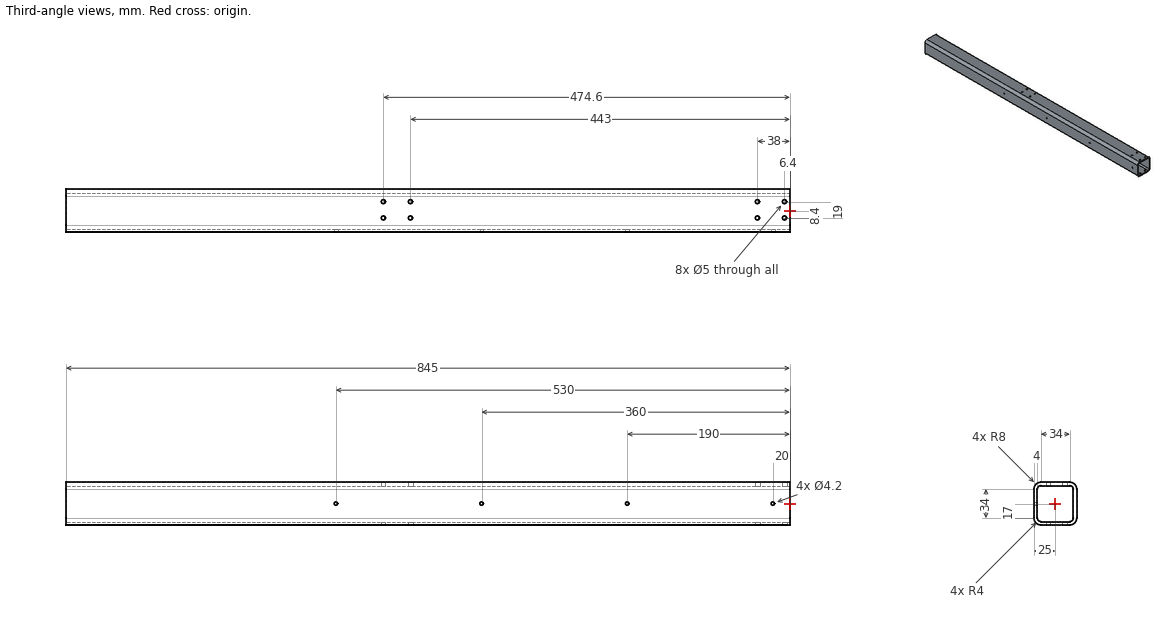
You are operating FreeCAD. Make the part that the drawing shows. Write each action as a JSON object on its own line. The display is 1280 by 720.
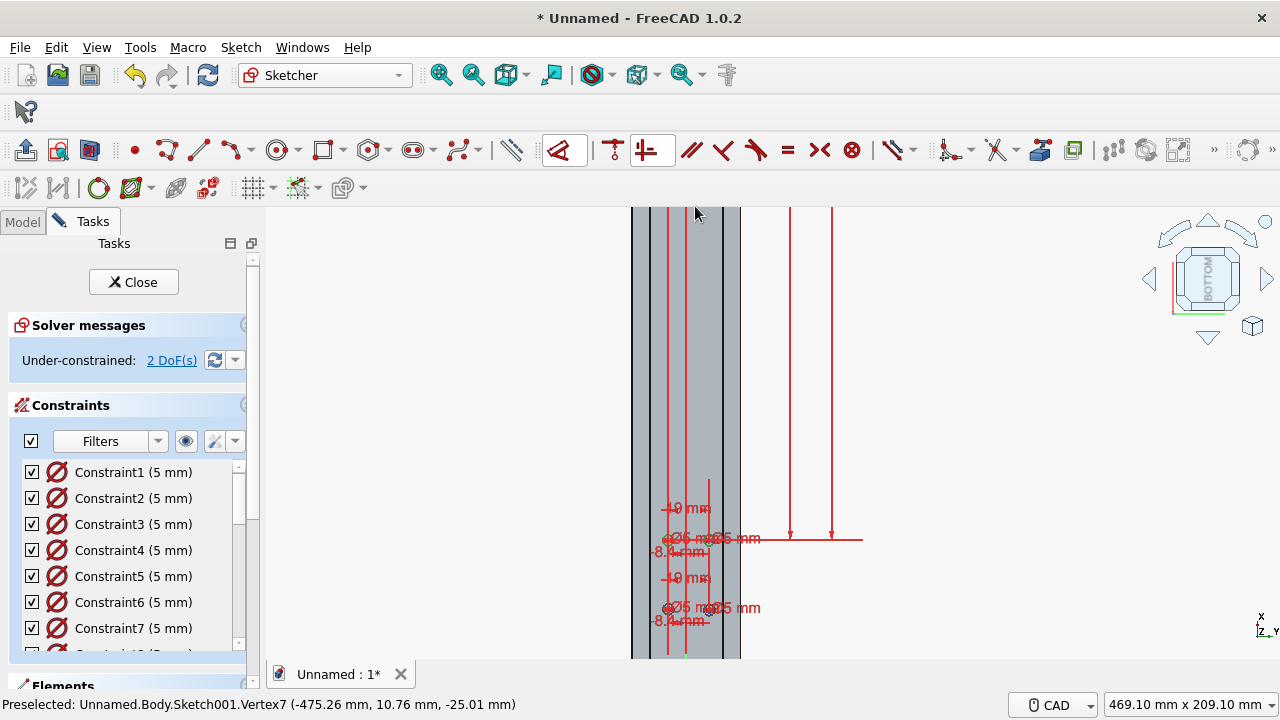
{"action": "scroll", "coordinate": [710, 542], "scroll_direction": "down", "scroll_amount": 7}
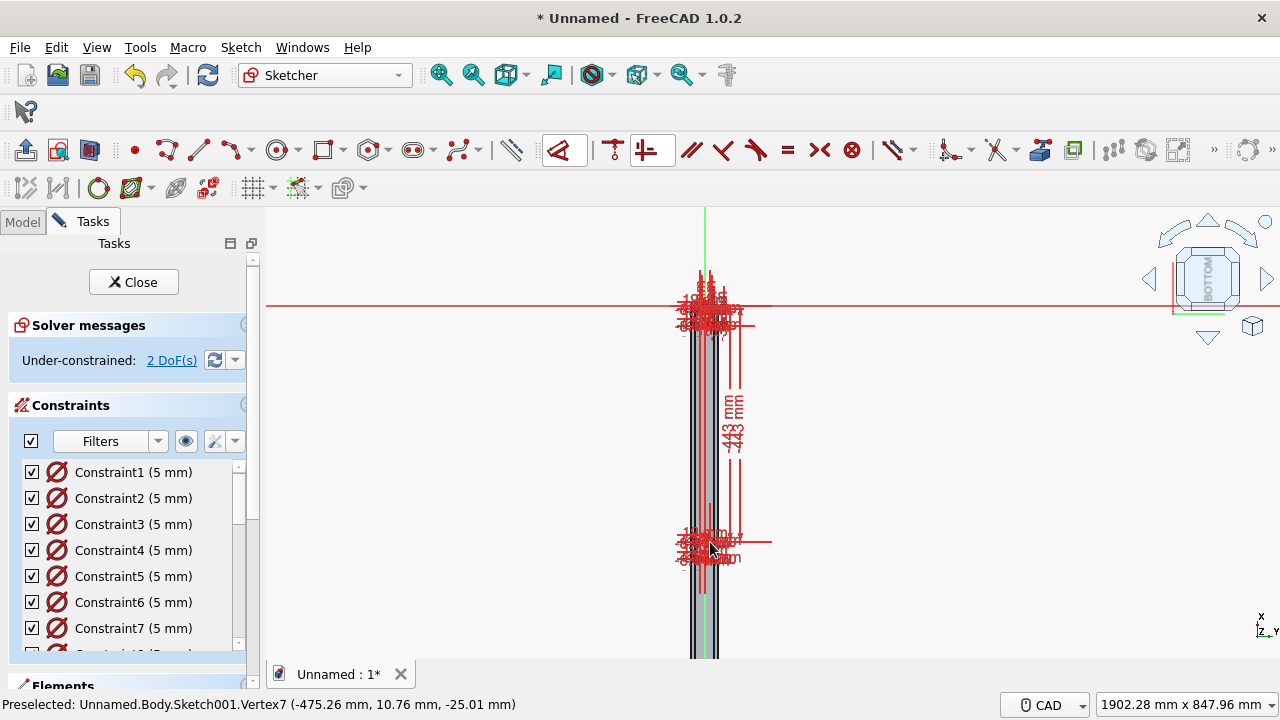
{"action": "left_click", "coordinate": [710, 559]}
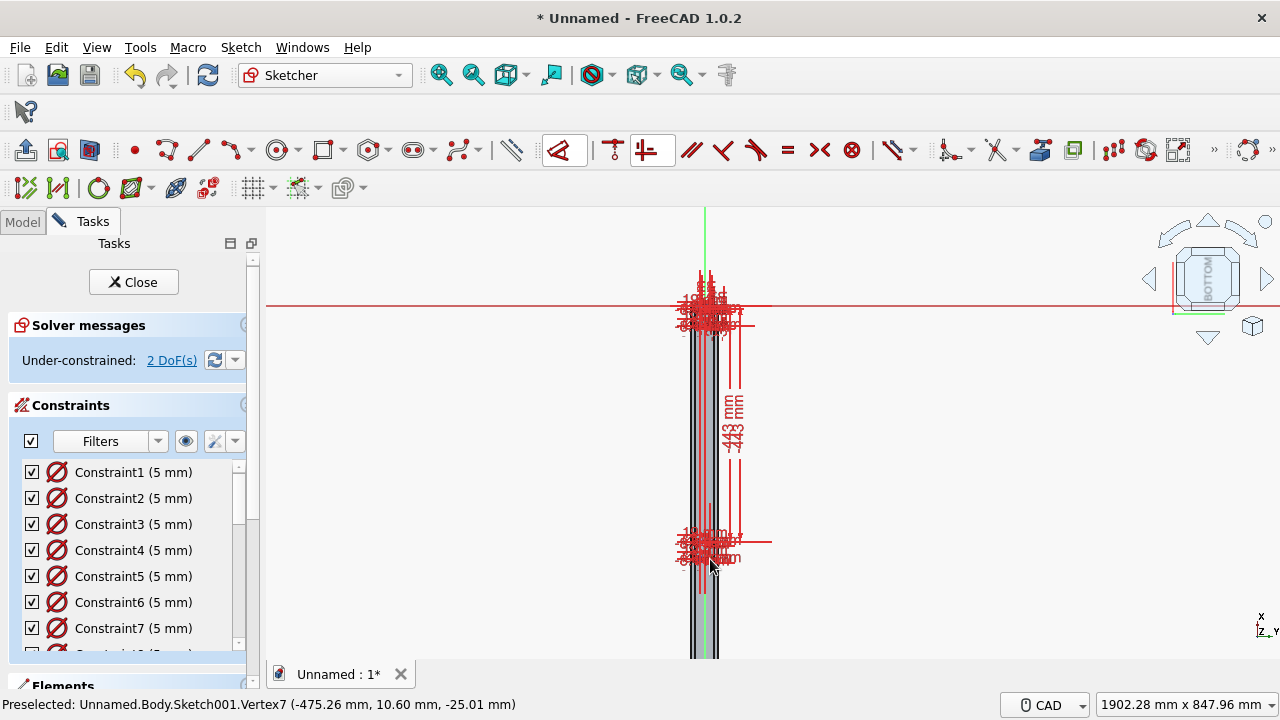
{"action": "key", "text": "i"}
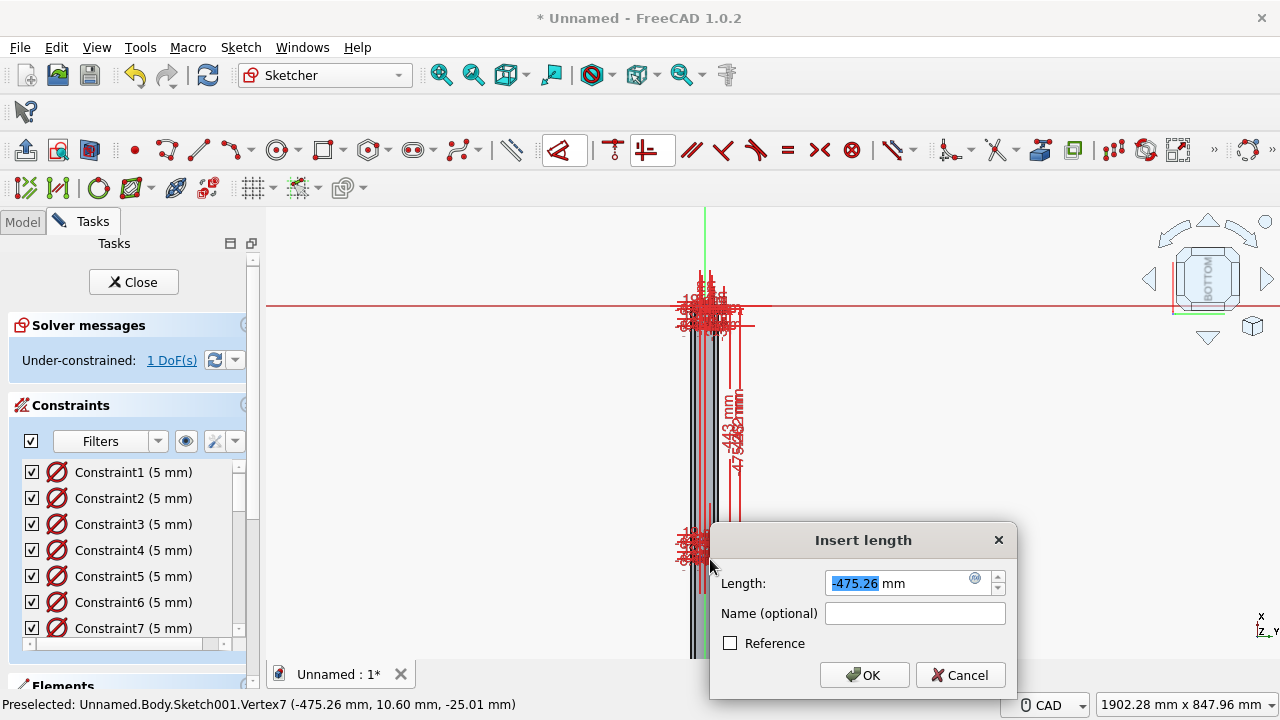
{"action": "type", "text": "-474.6"}
{"action": "key", "text": "Return"}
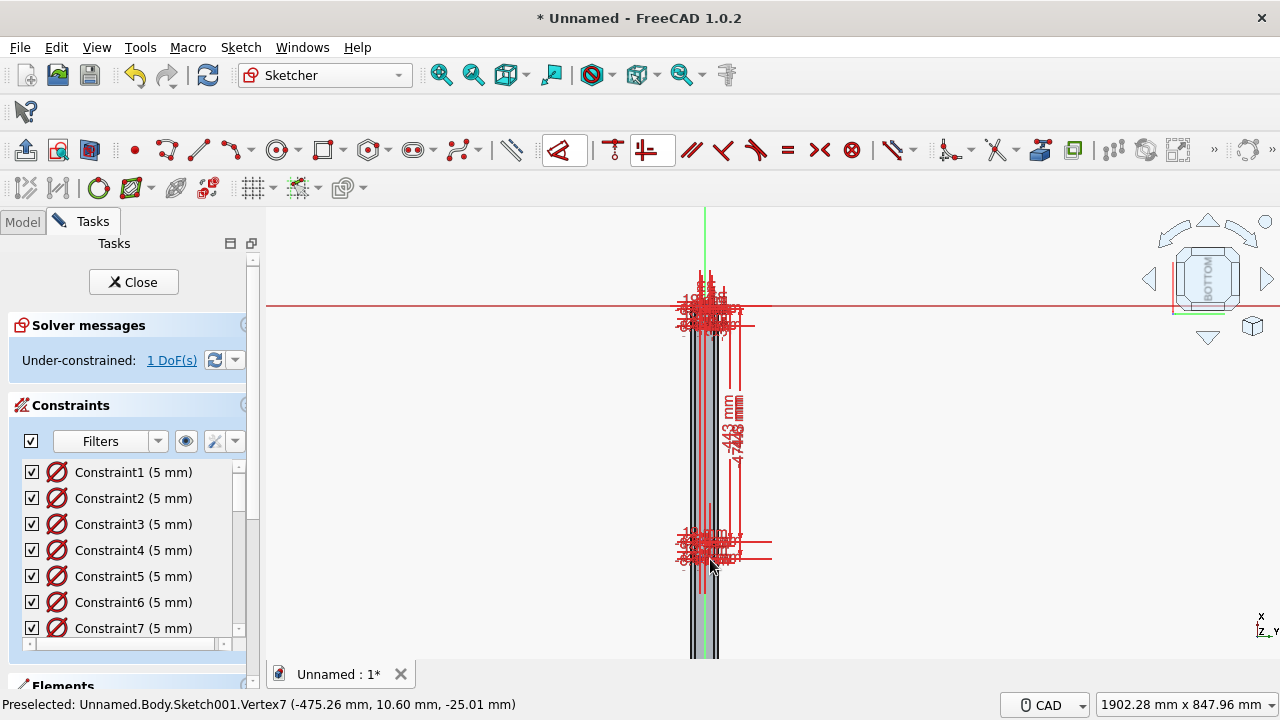
{"action": "left_click", "coordinate": [700, 559]}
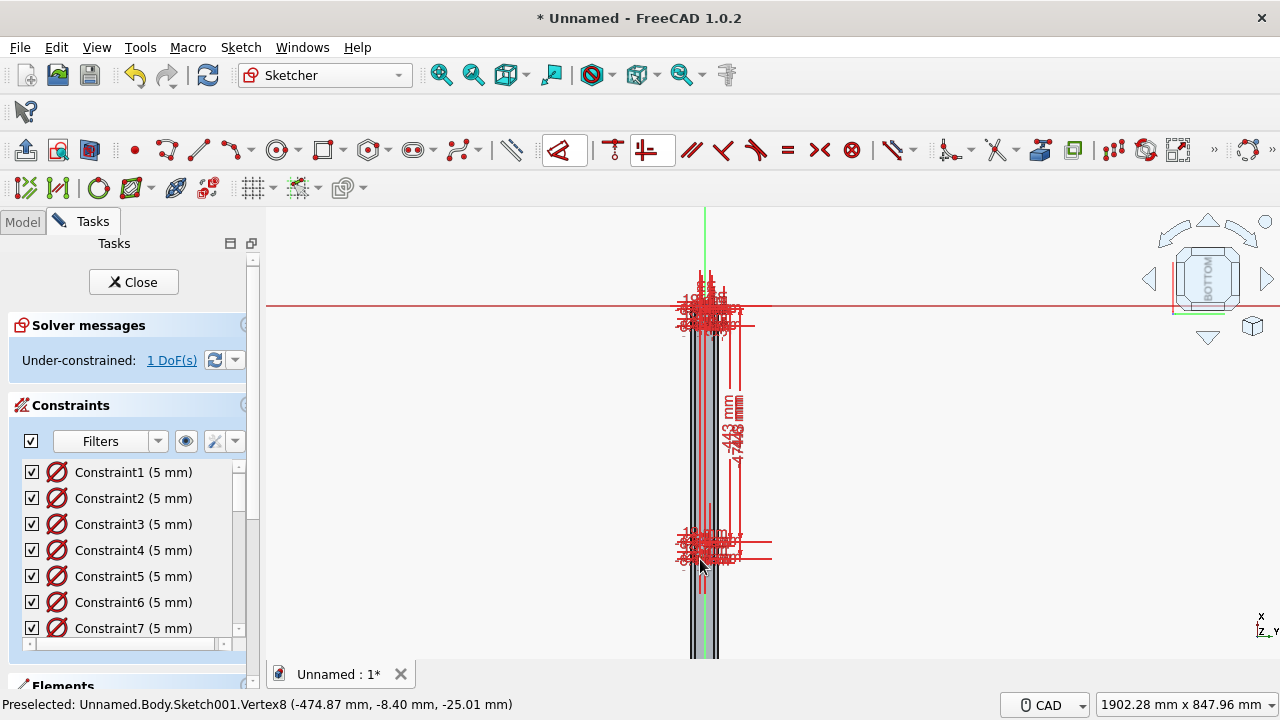
{"action": "left_click", "coordinate": [582, 150]}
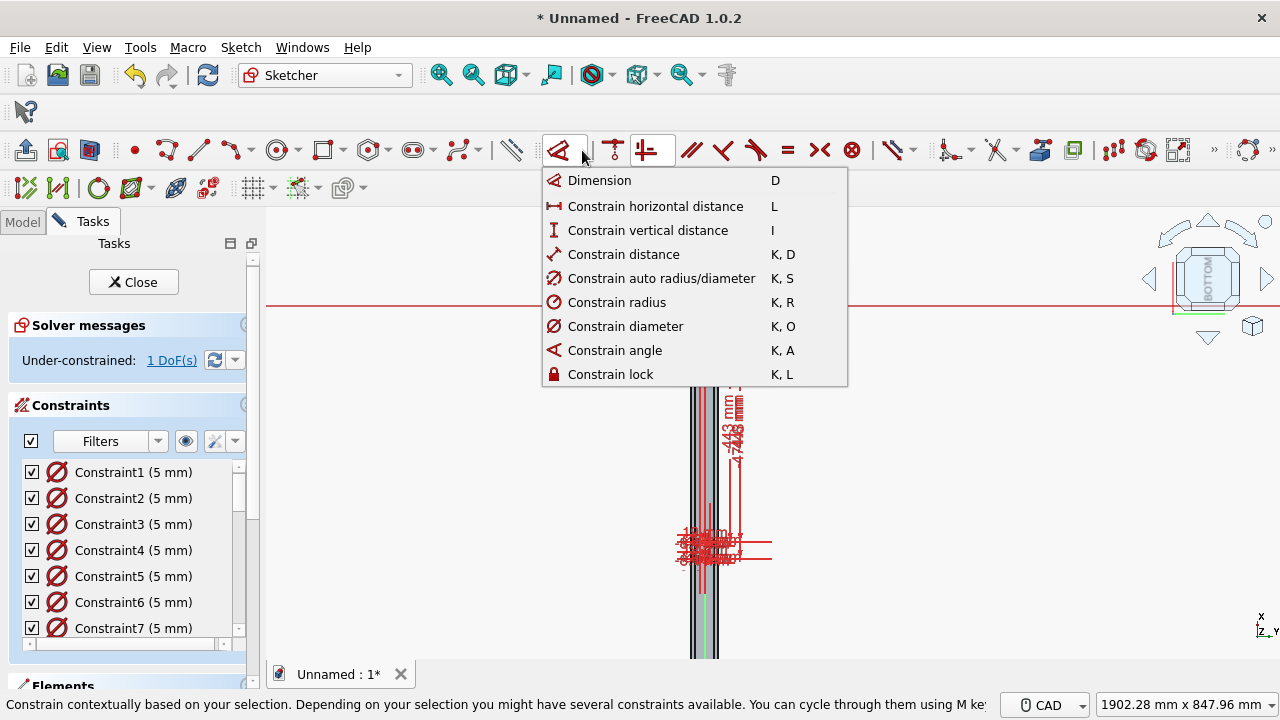
{"action": "left_click", "coordinate": [695, 230]}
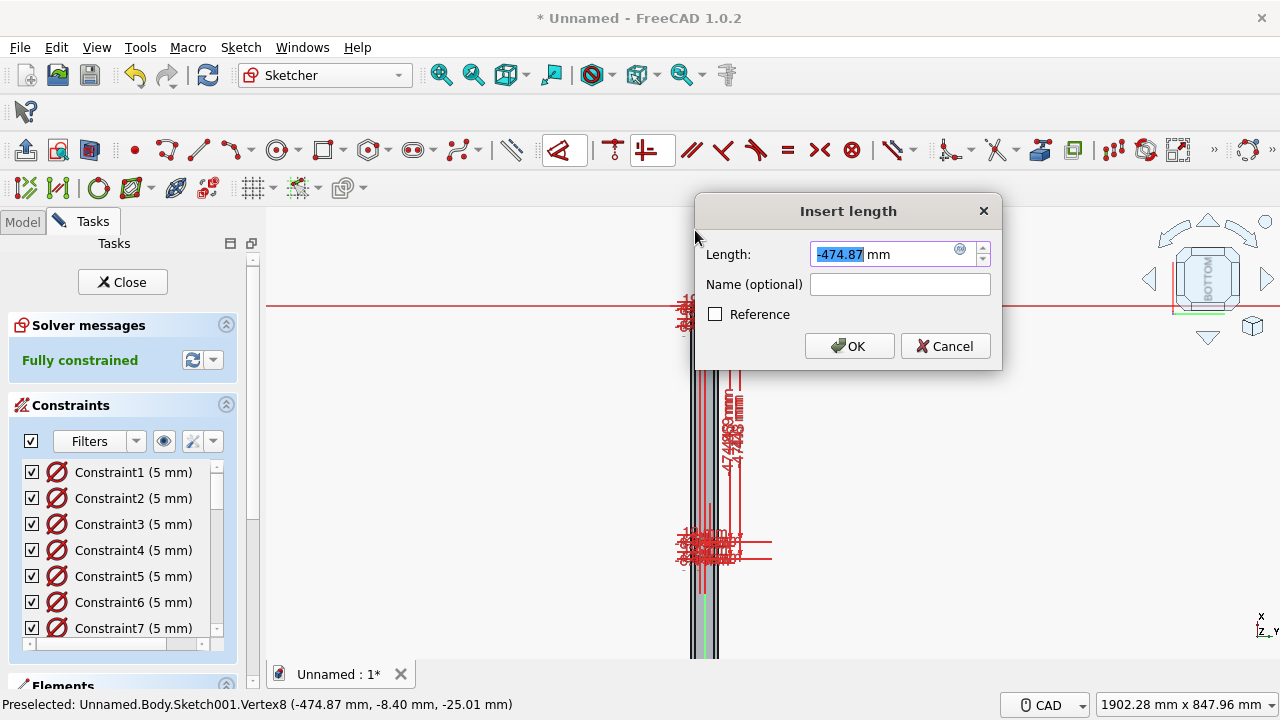
{"action": "type", "text": "-474.6"}
{"action": "key", "text": "Return"}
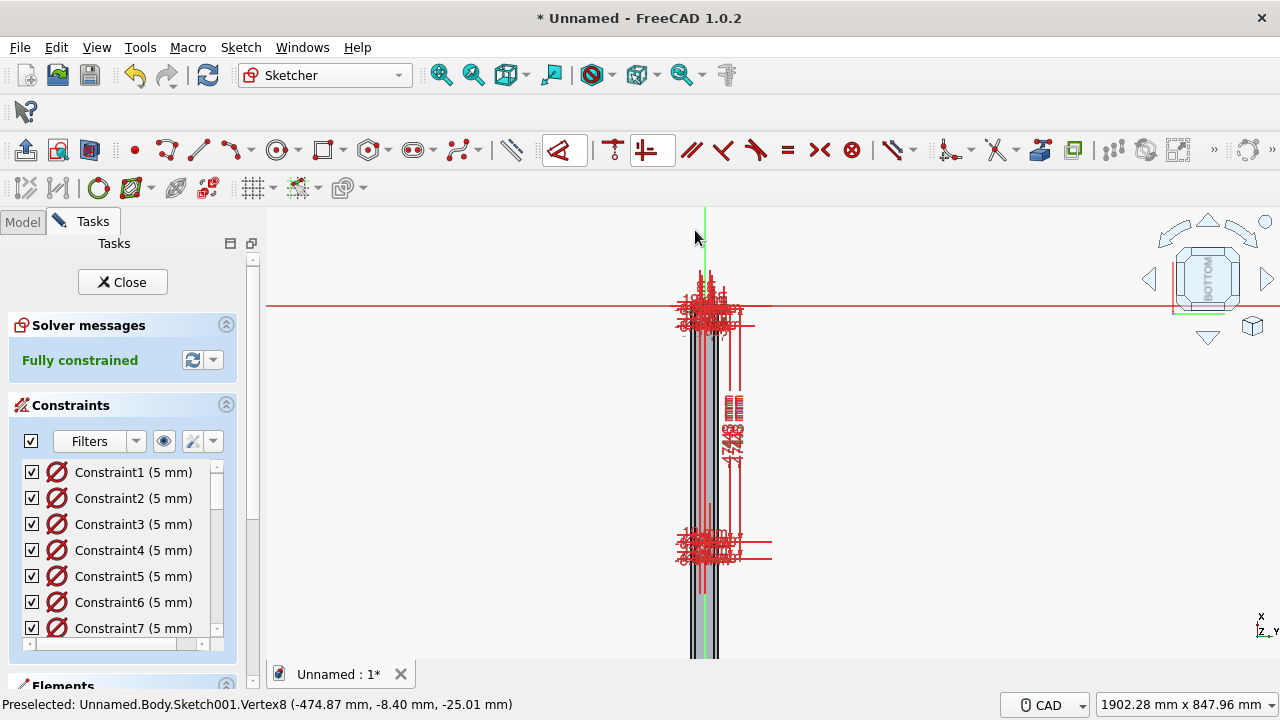
{"action": "left_click", "coordinate": [123, 282]}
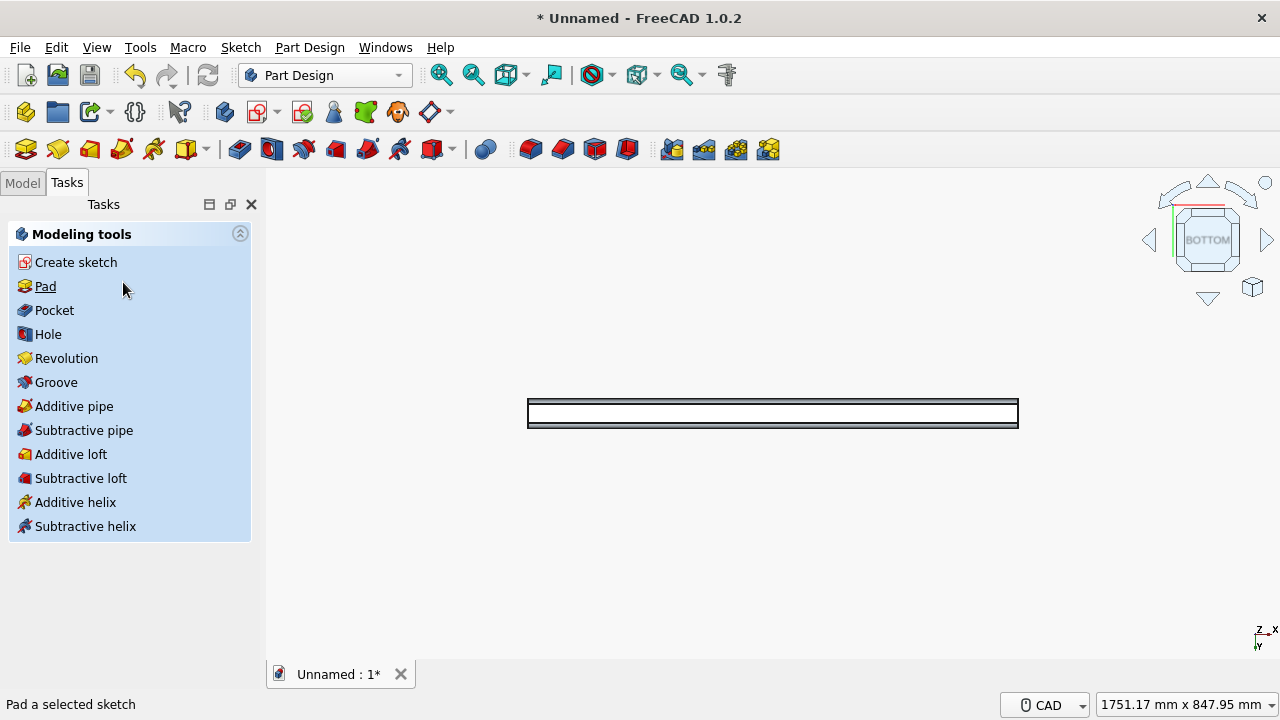
{"action": "left_click", "coordinate": [272, 150]}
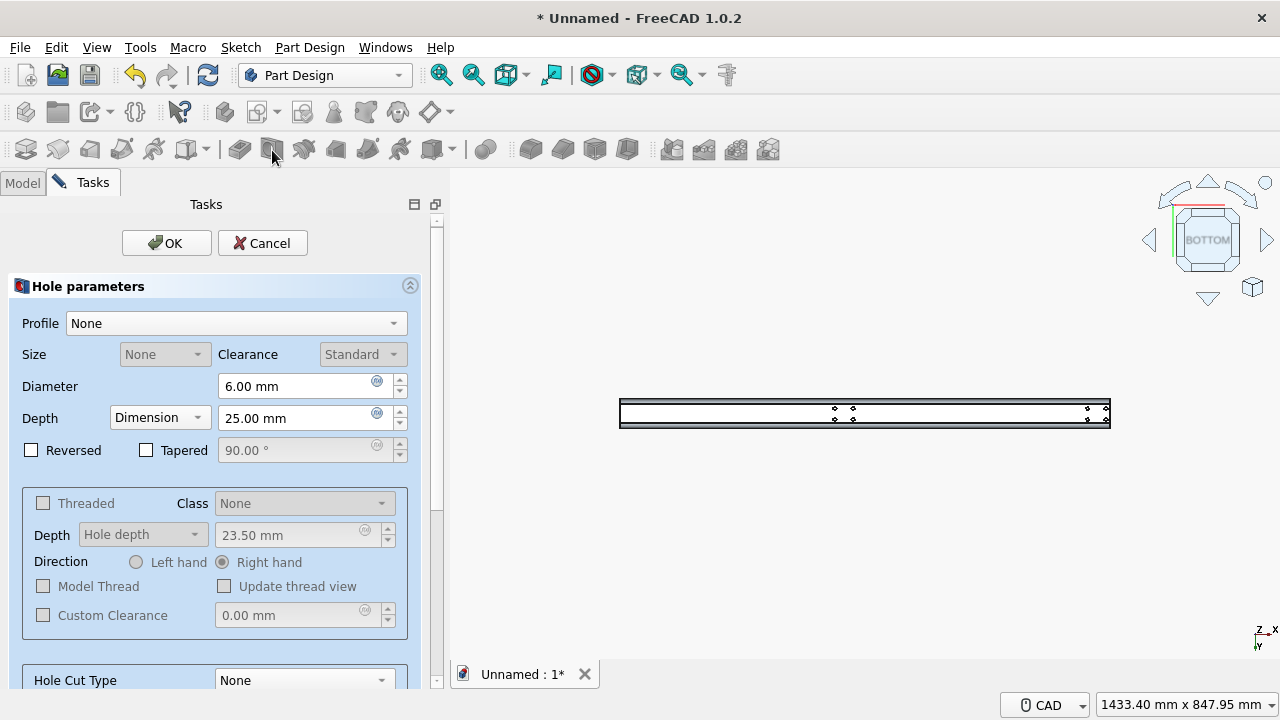
{"action": "triple_click", "coordinate": [305, 386]}